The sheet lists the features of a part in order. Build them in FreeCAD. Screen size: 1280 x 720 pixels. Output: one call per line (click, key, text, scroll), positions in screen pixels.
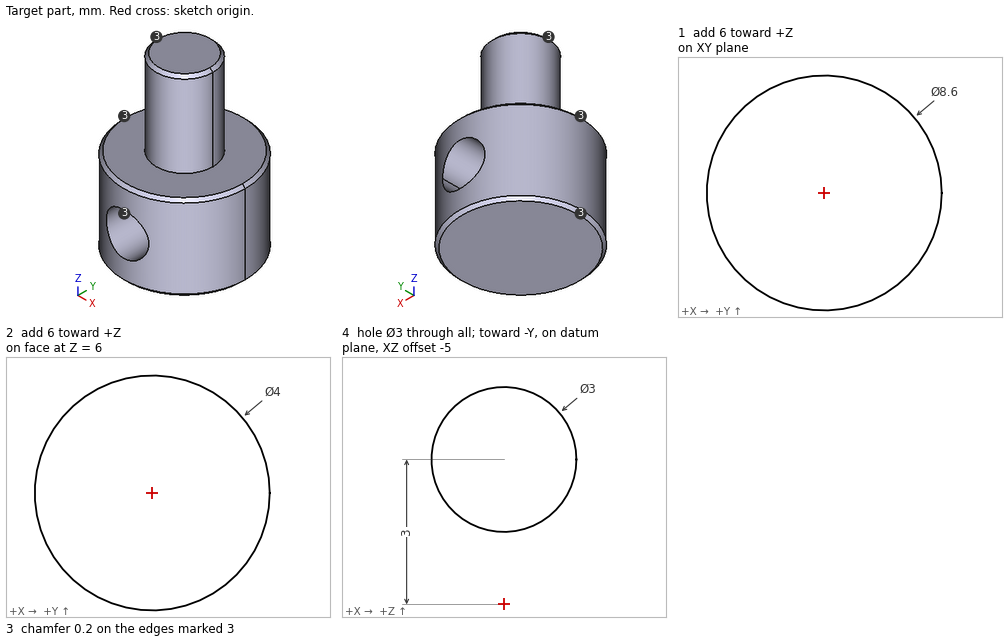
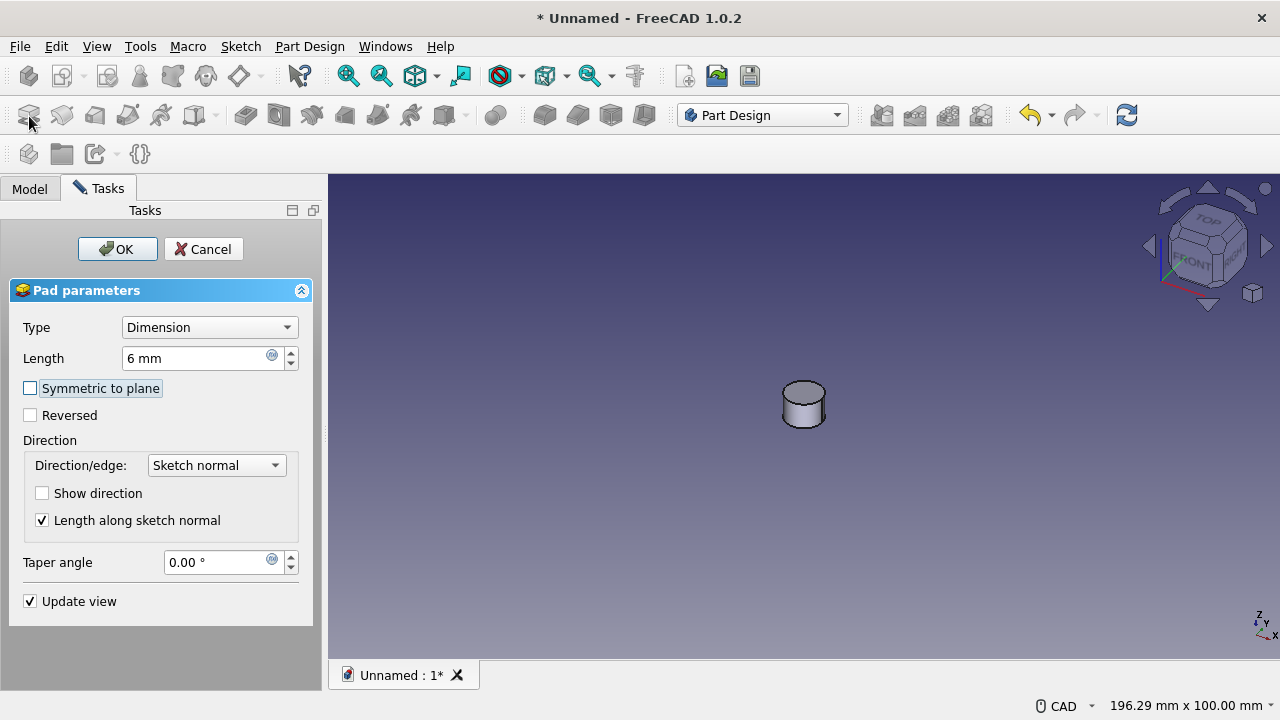
click(118, 249)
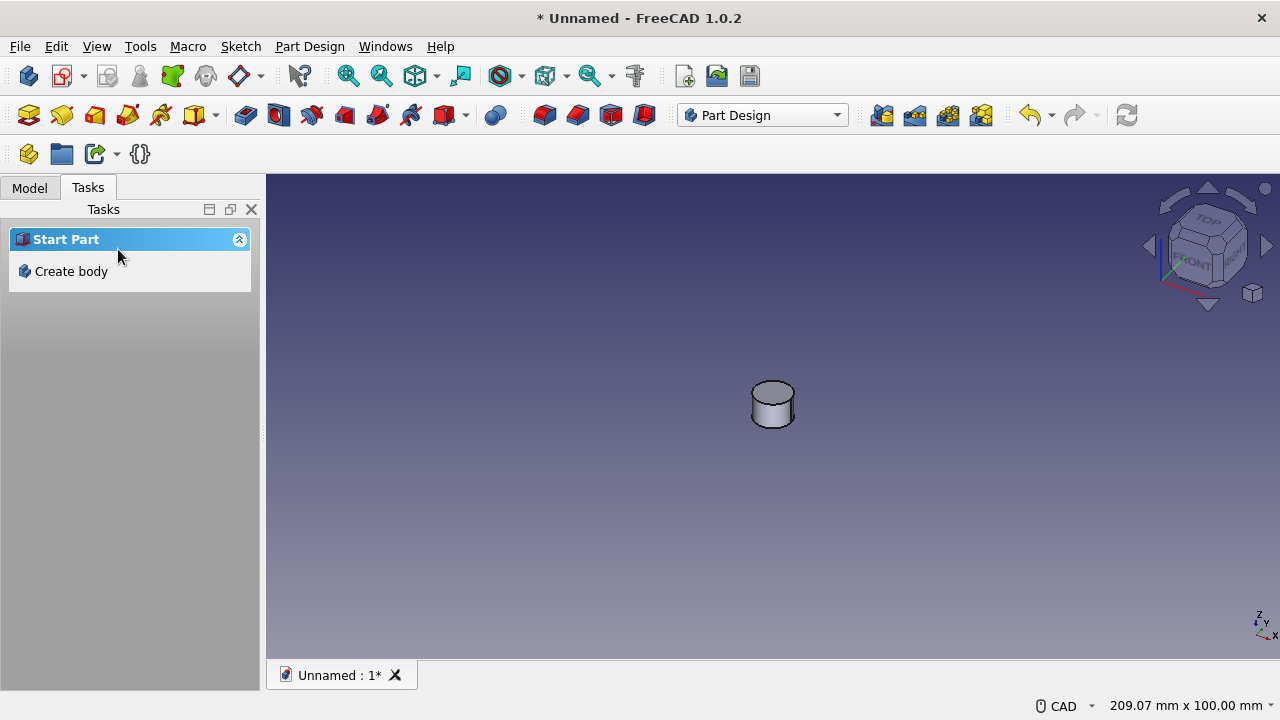
key(v)
key(f)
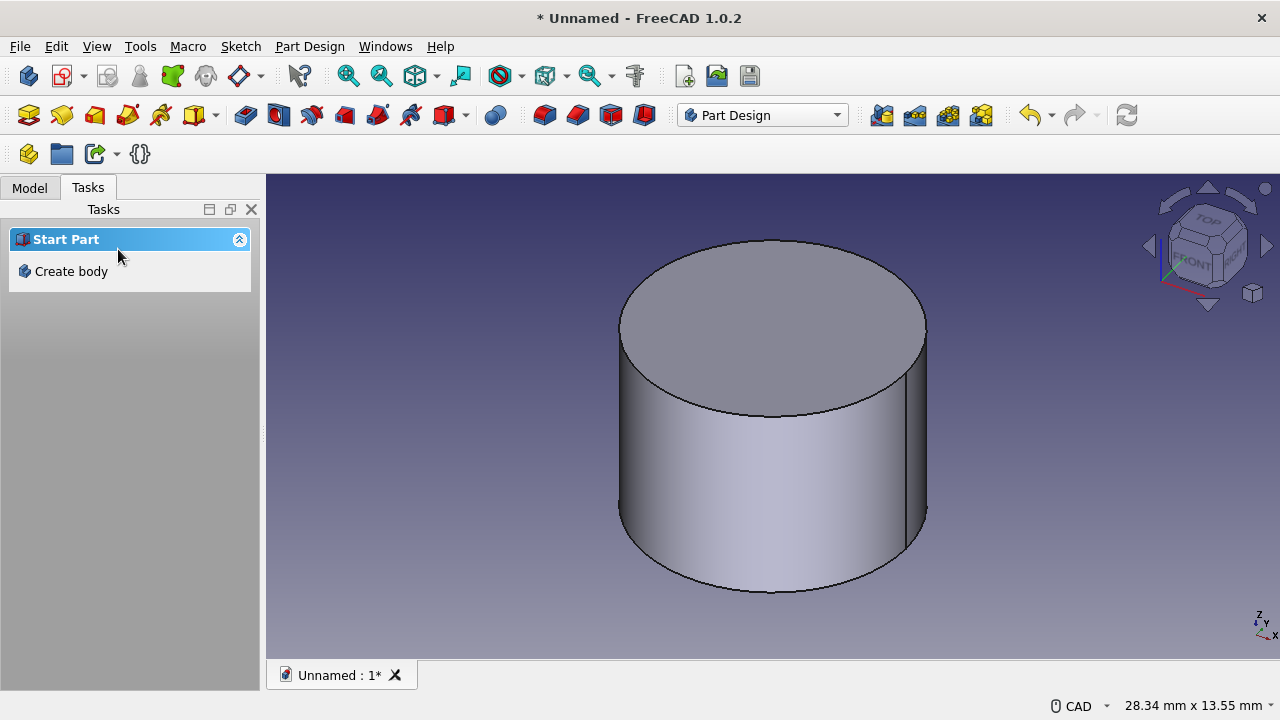
click(773, 328)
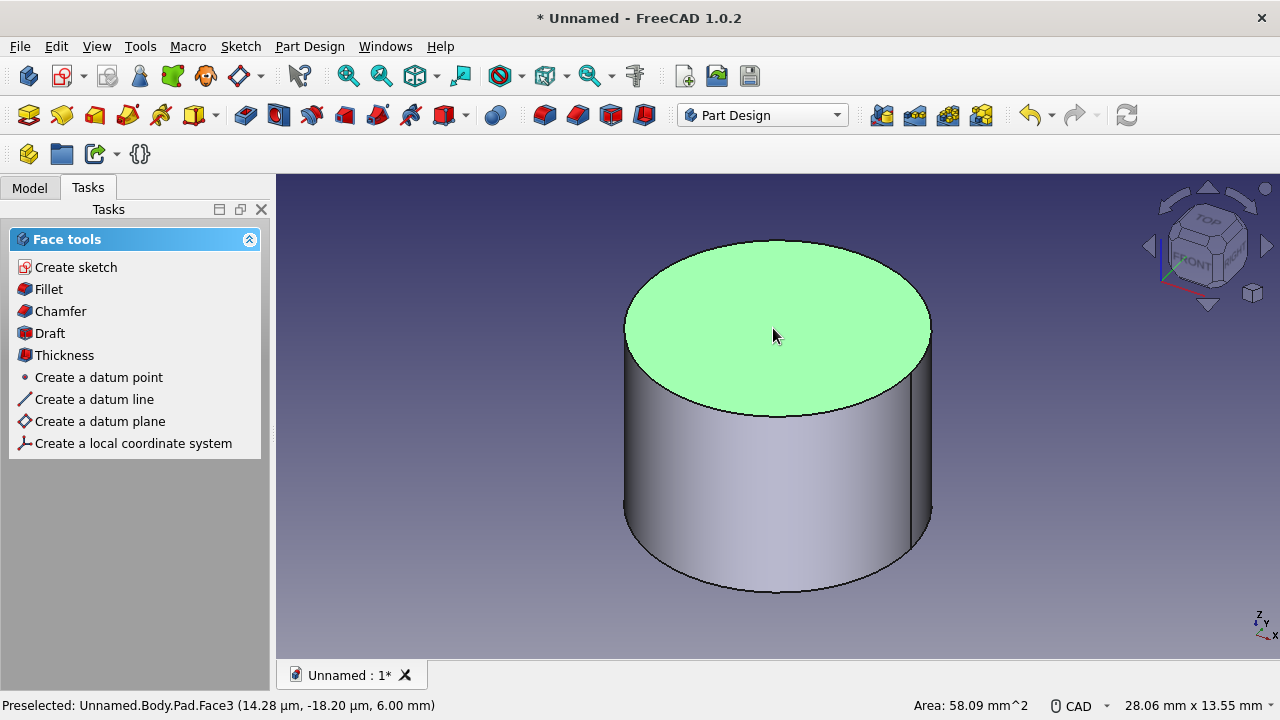
click(62, 76)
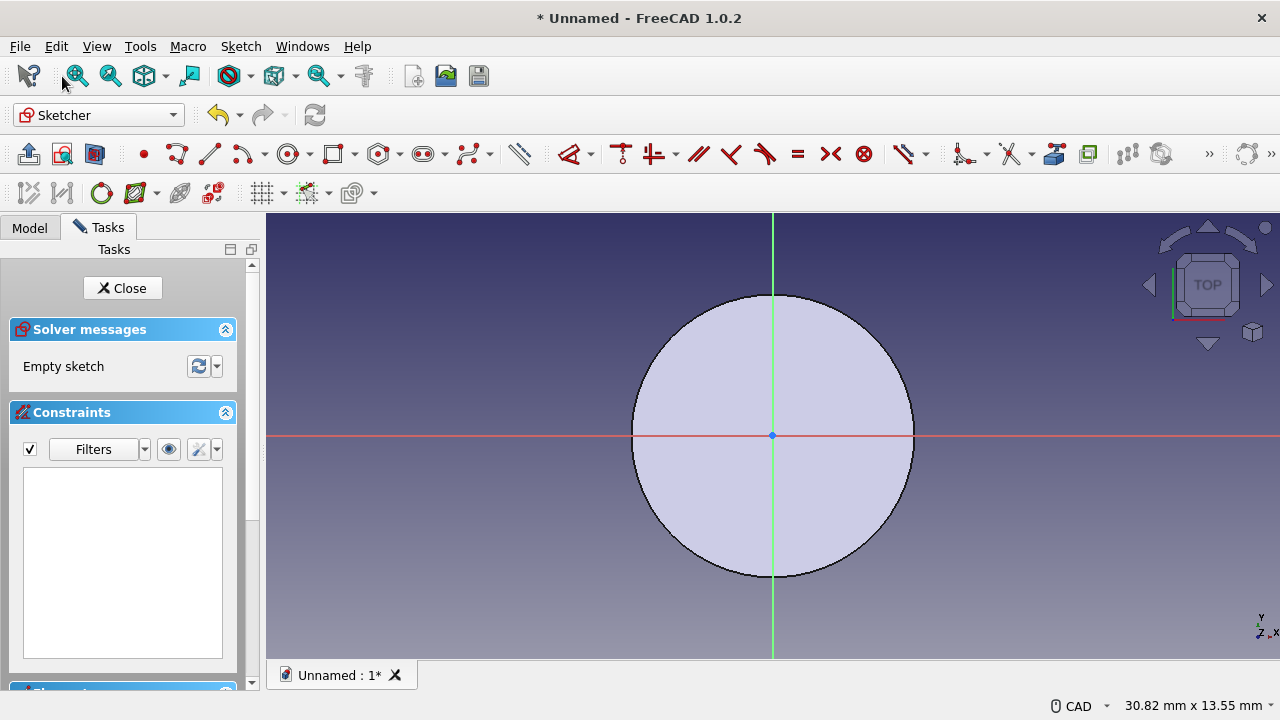
scroll(829, 436, up, 4)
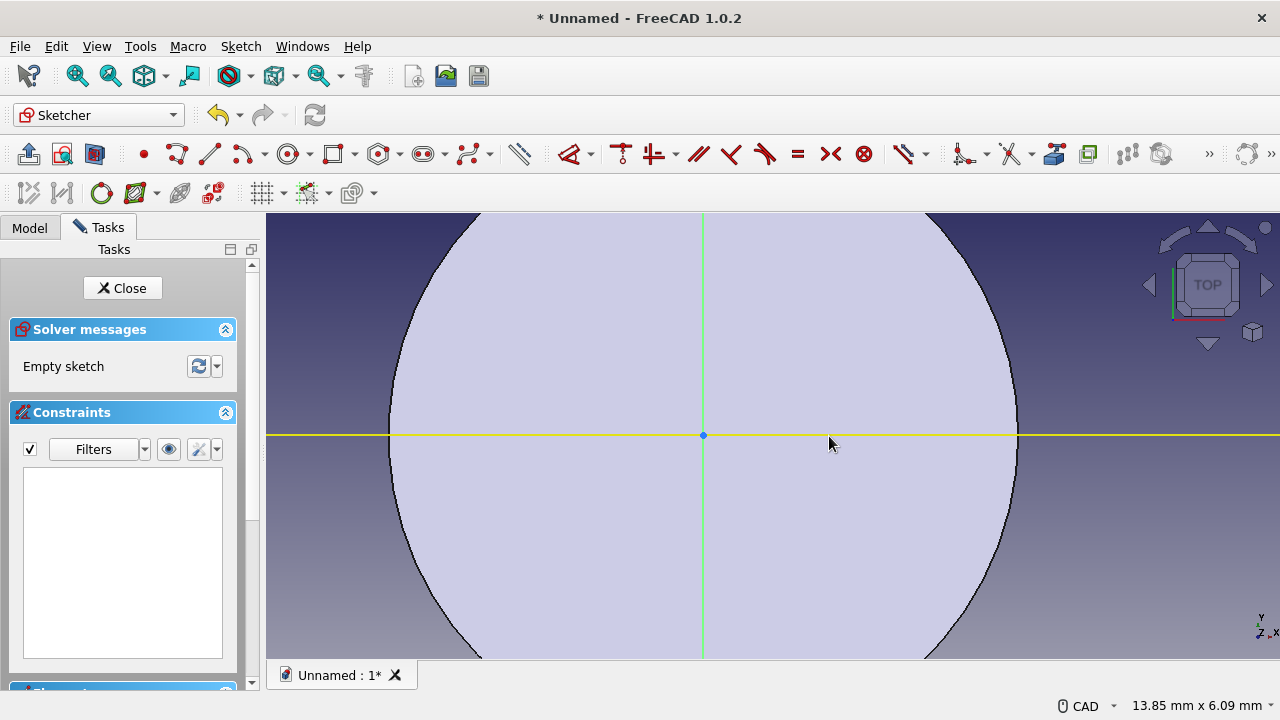
key(g)
key(c)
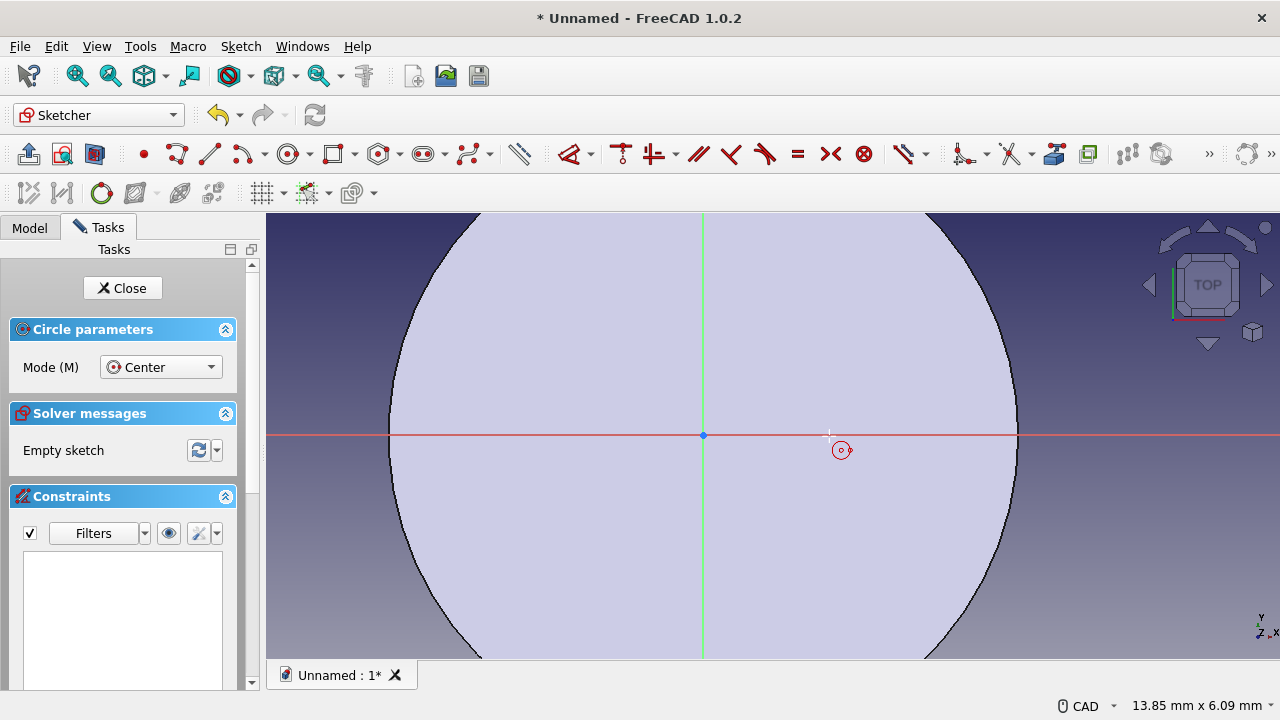
click(703, 435)
move(807, 332)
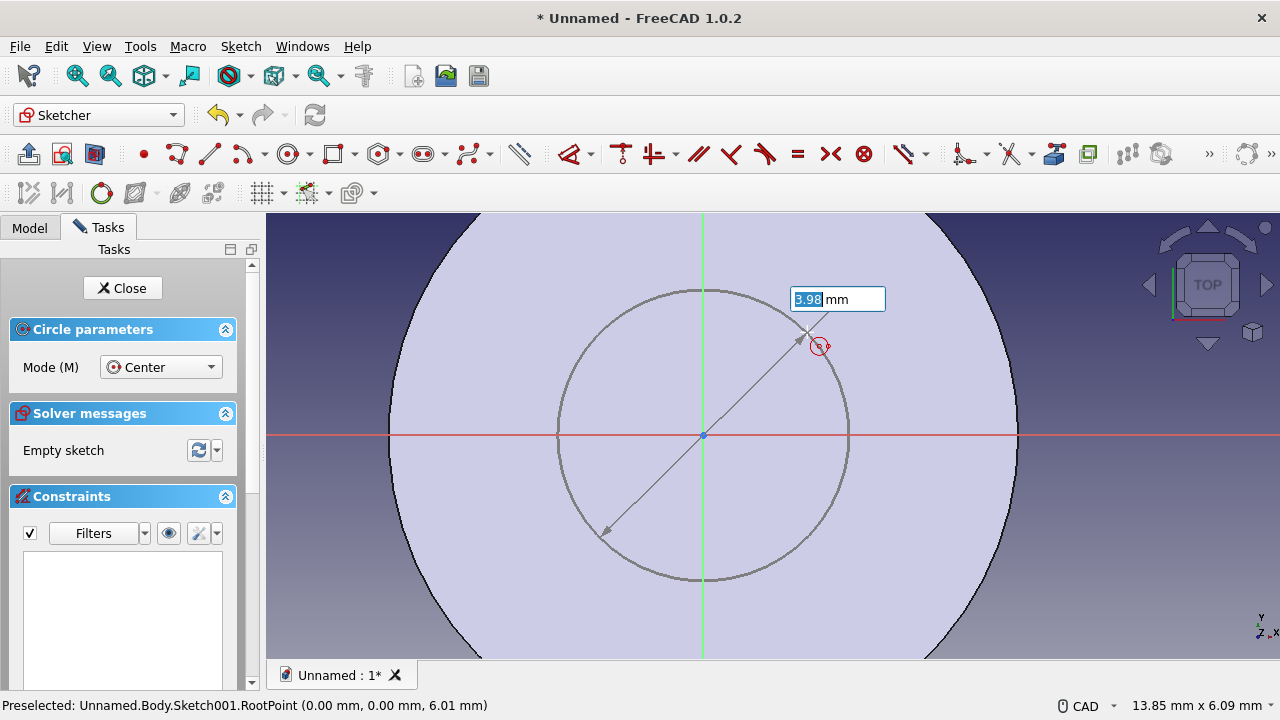
text(4)
key(Return)
key(Escape)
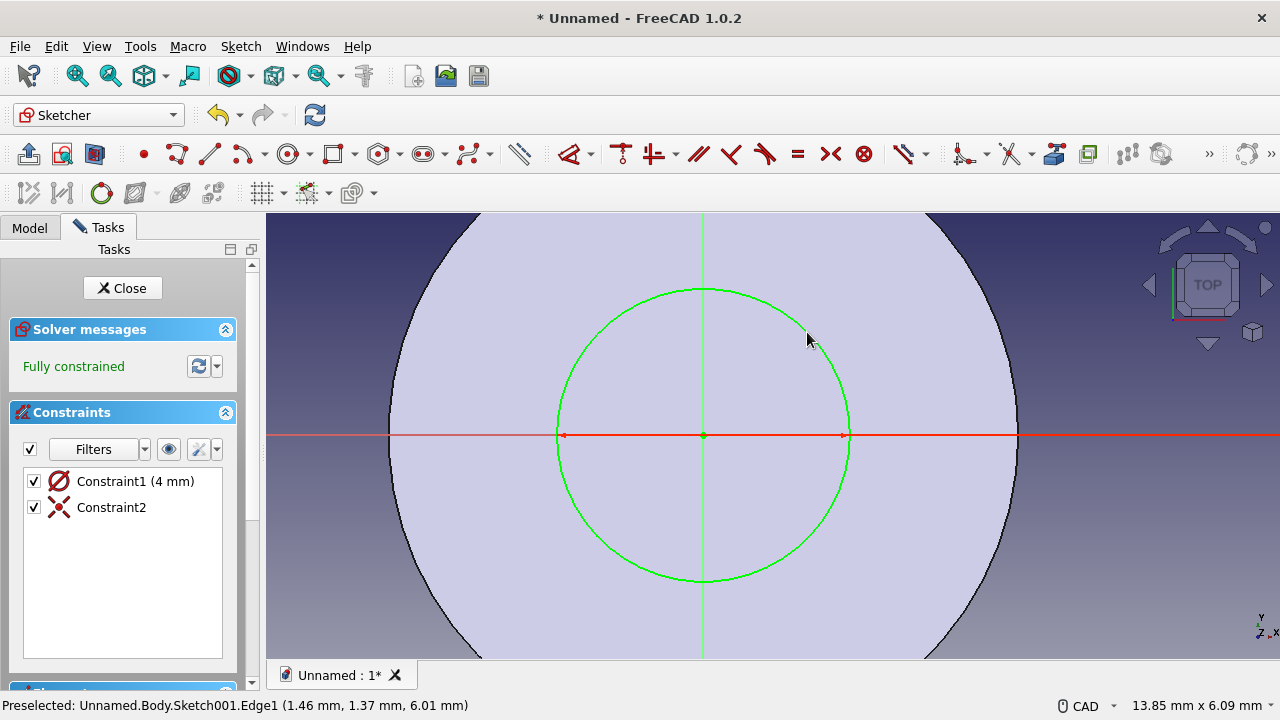
click(123, 288)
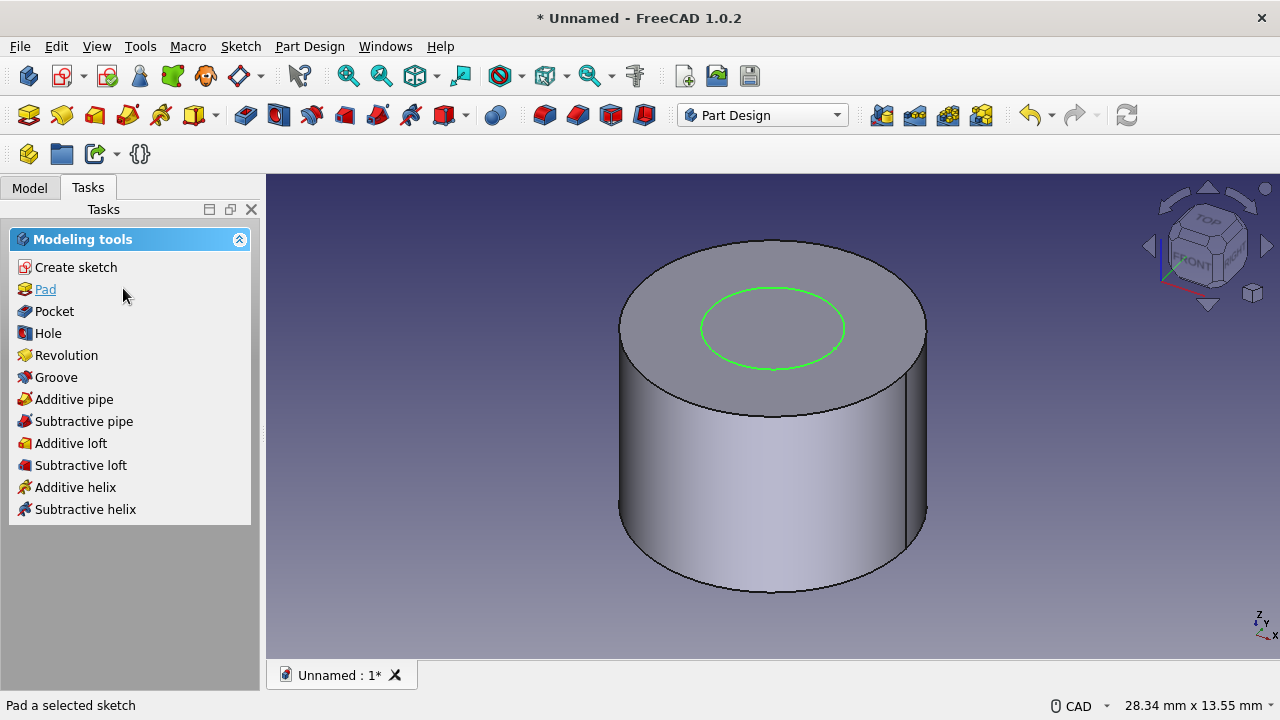
click(29, 116)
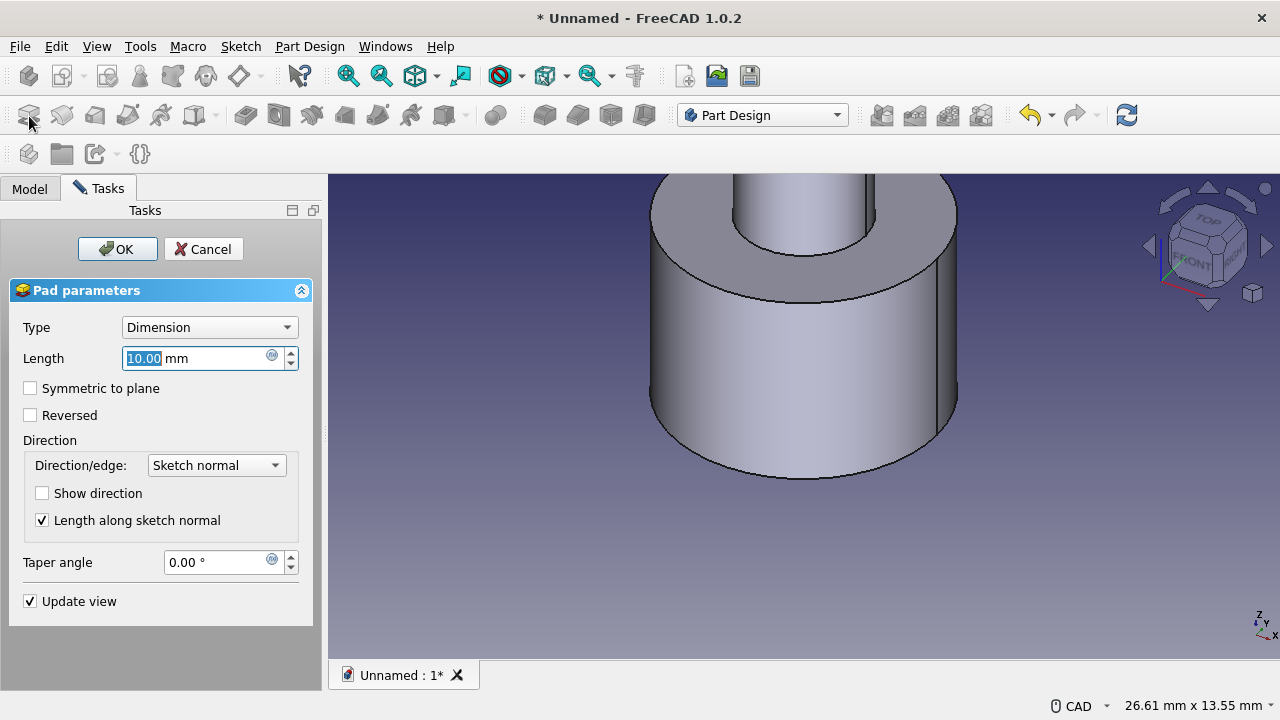
text(6)
key(Tab)